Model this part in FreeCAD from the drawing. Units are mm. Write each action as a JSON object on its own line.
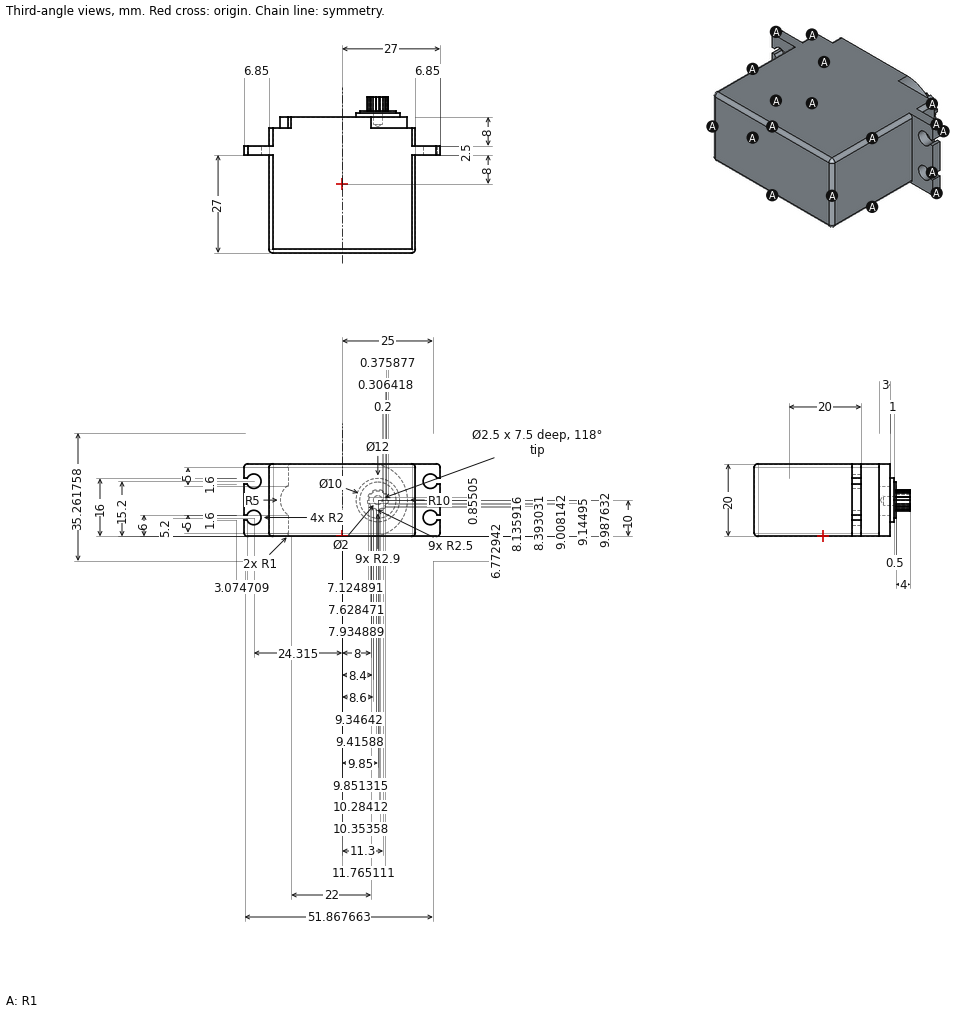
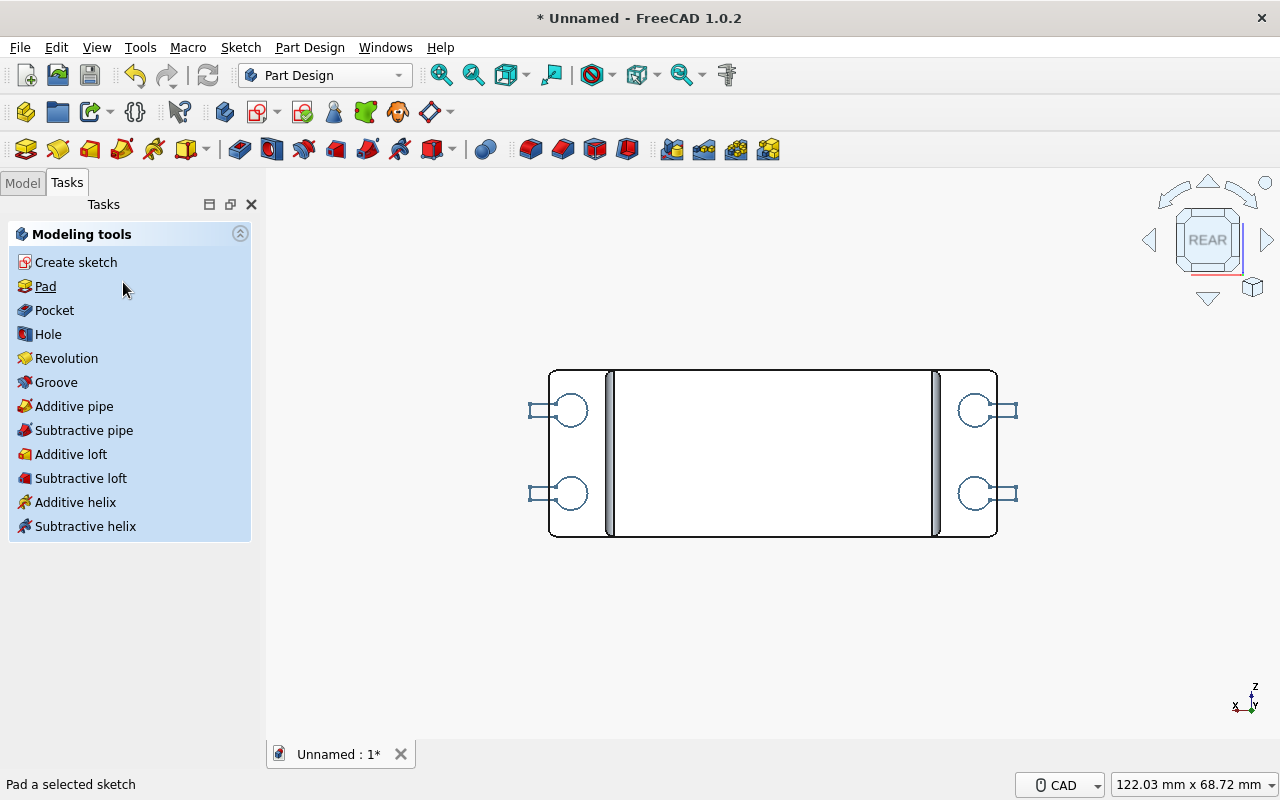
{"action": "left_click", "coordinate": [240, 150]}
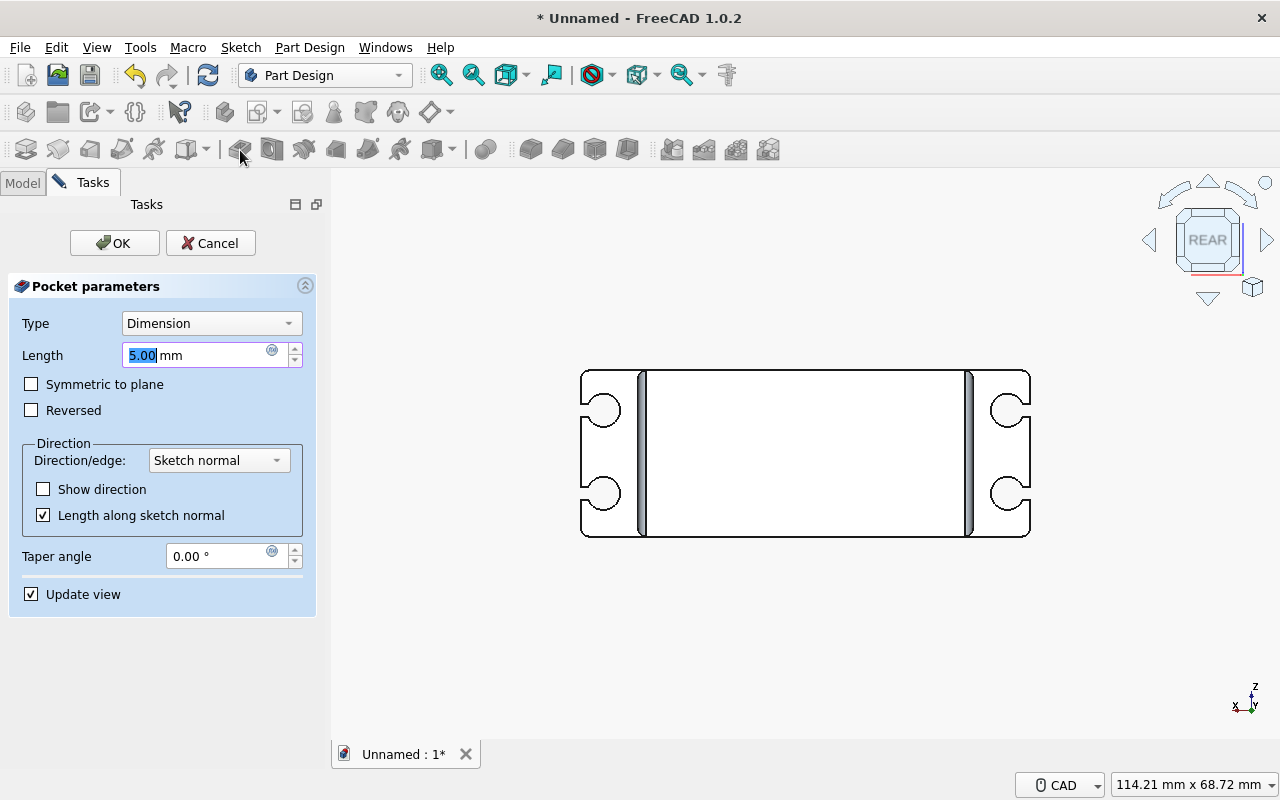
{"action": "type", "text": "20"}
{"action": "key", "text": "Tab"}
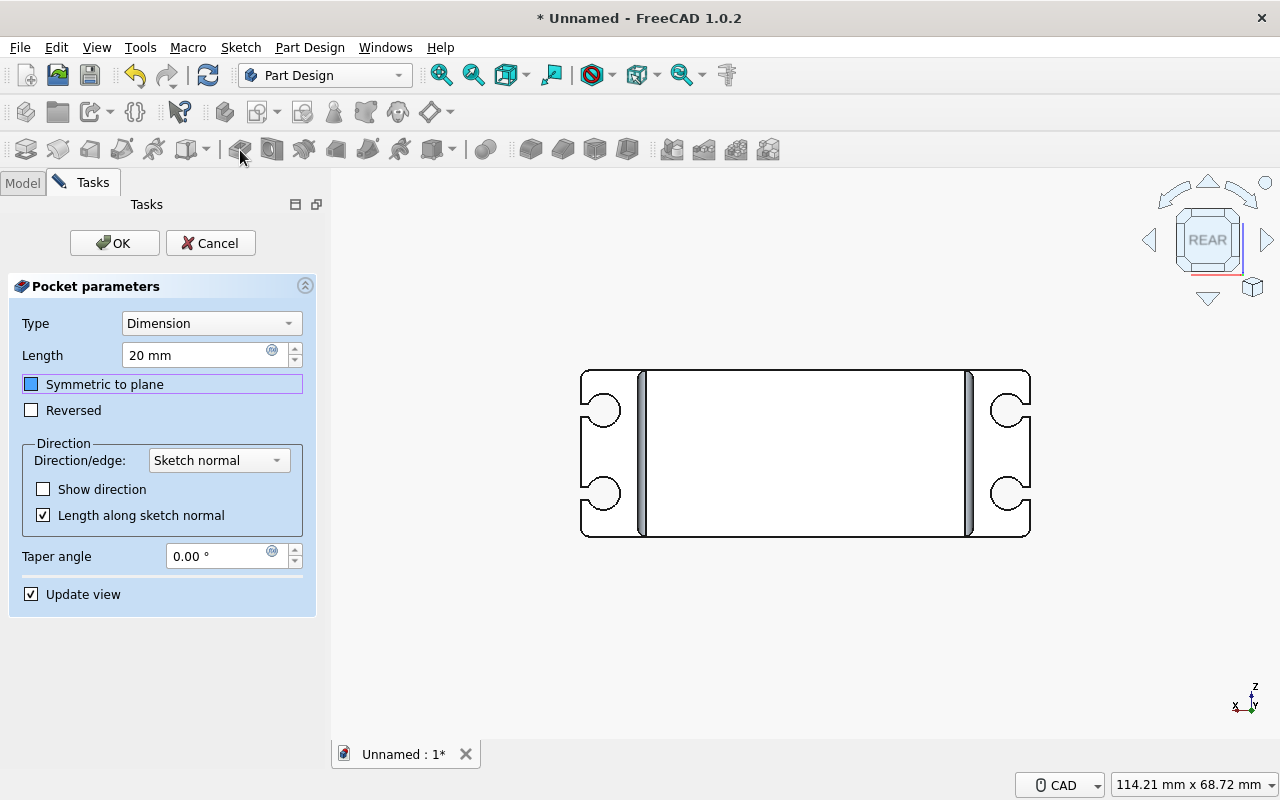
{"action": "left_click", "coordinate": [115, 243]}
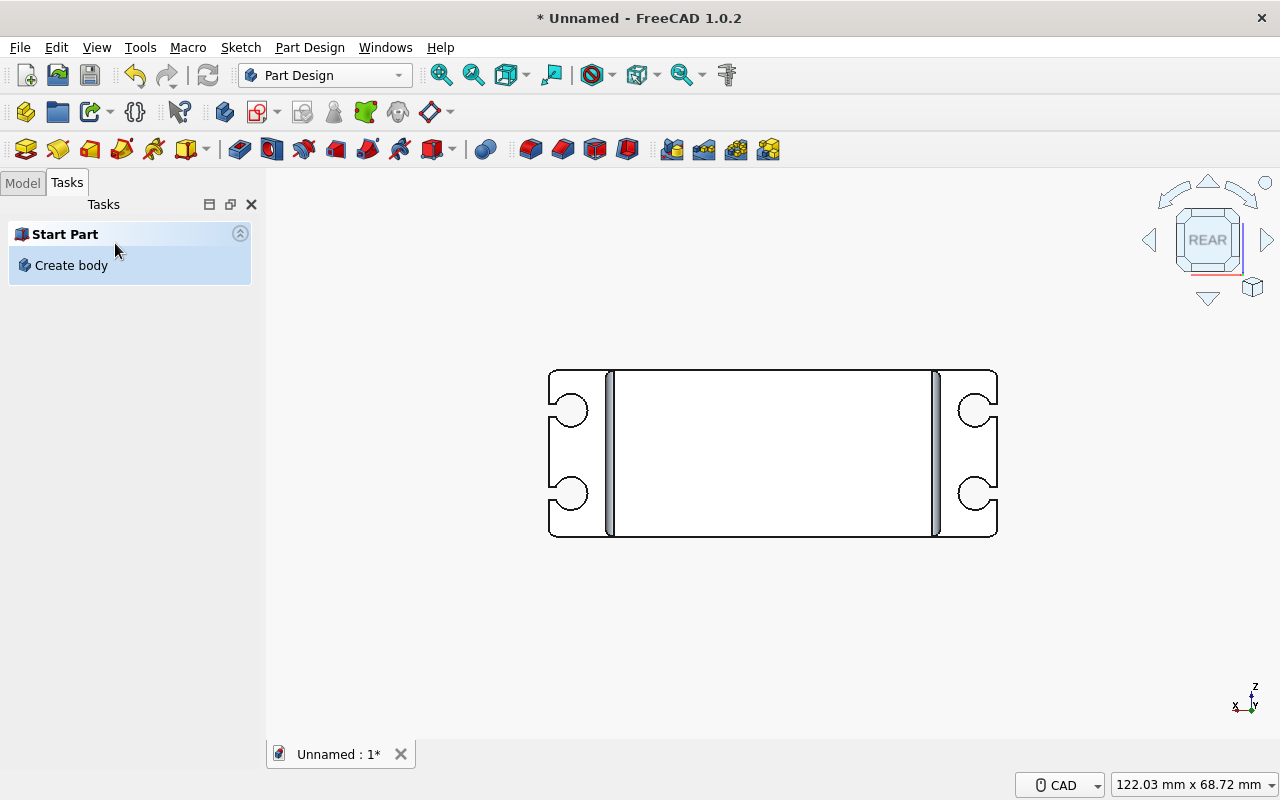
{"action": "left_click", "coordinate": [442, 76]}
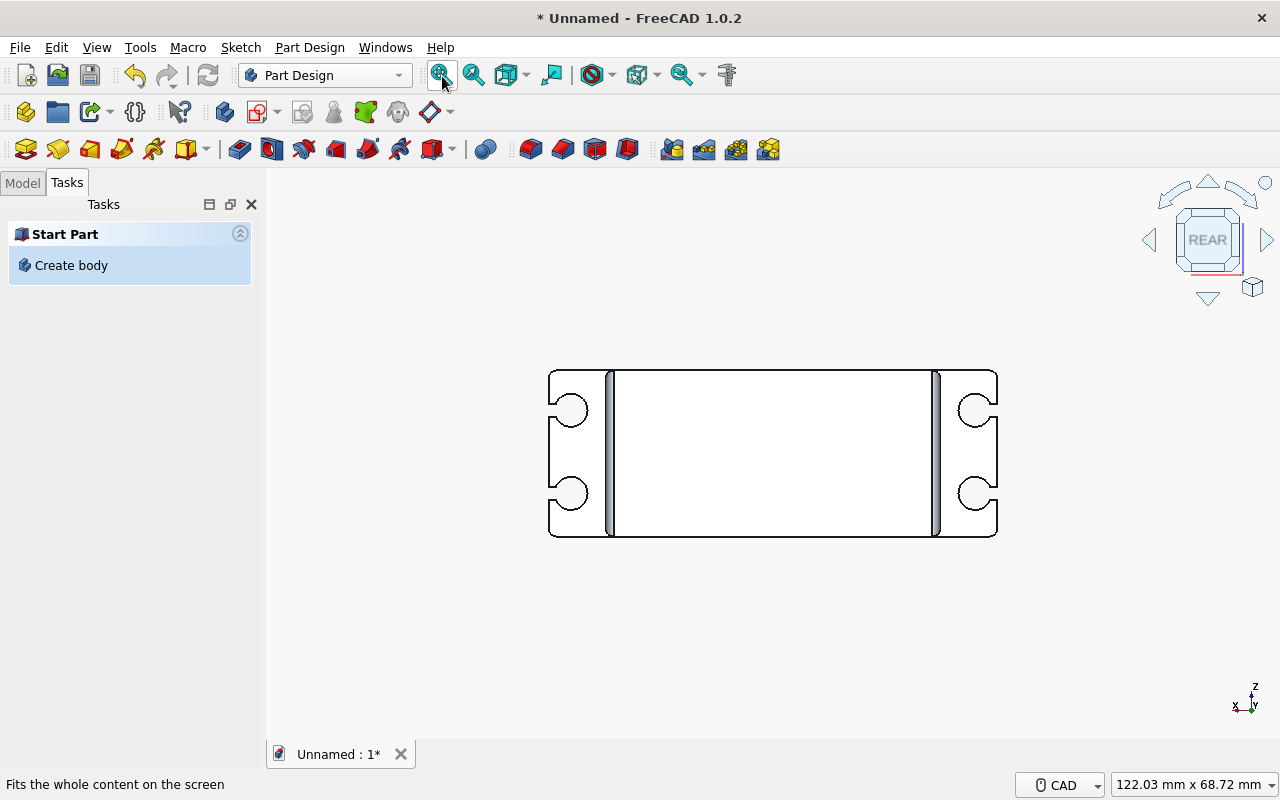
{"action": "left_click", "coordinate": [728, 452]}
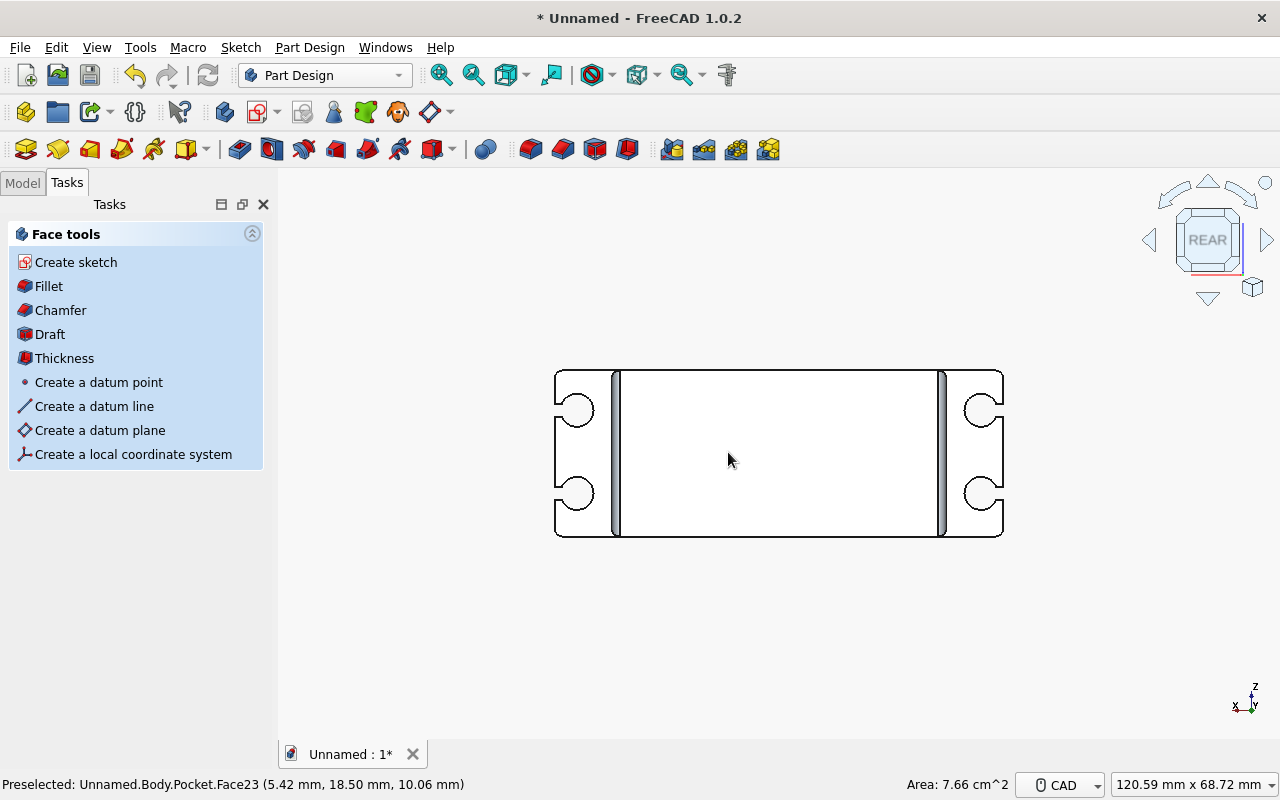
{"action": "left_click", "coordinate": [258, 112]}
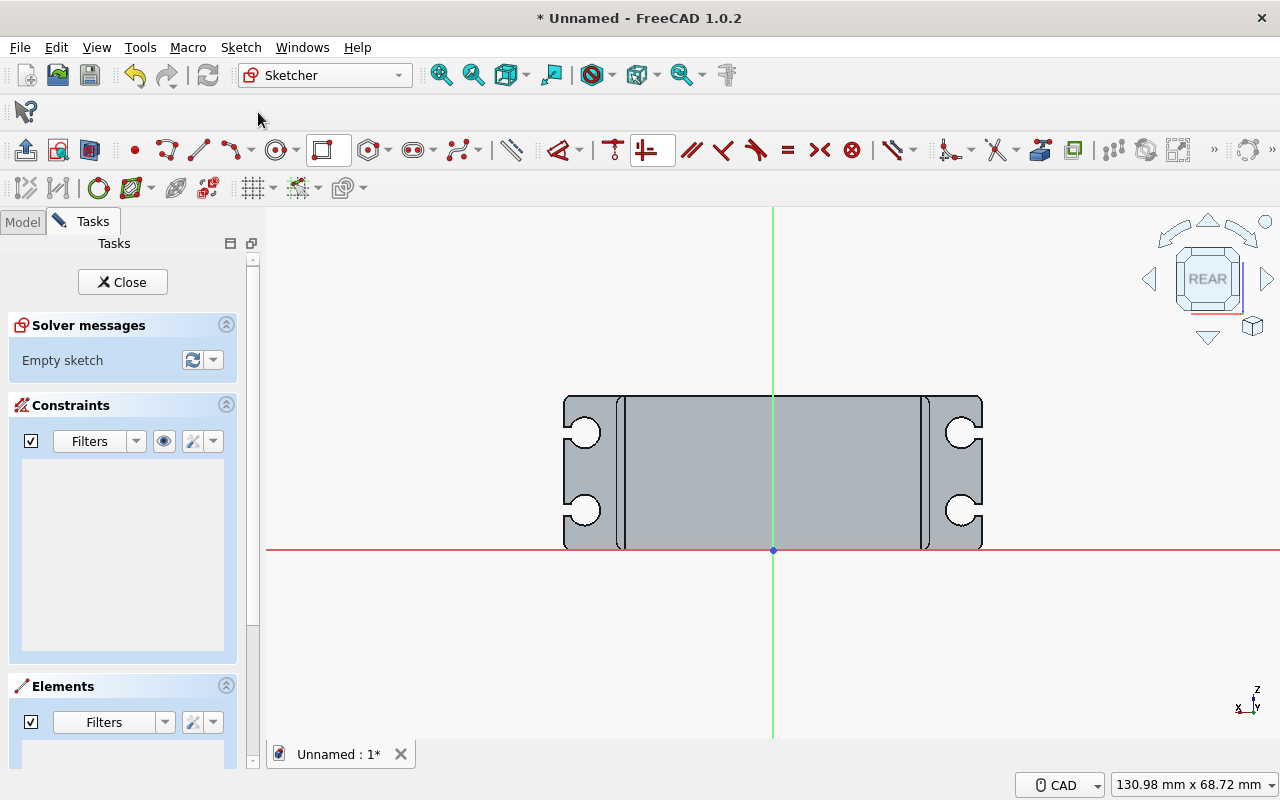
{"action": "left_click", "coordinate": [322, 150]}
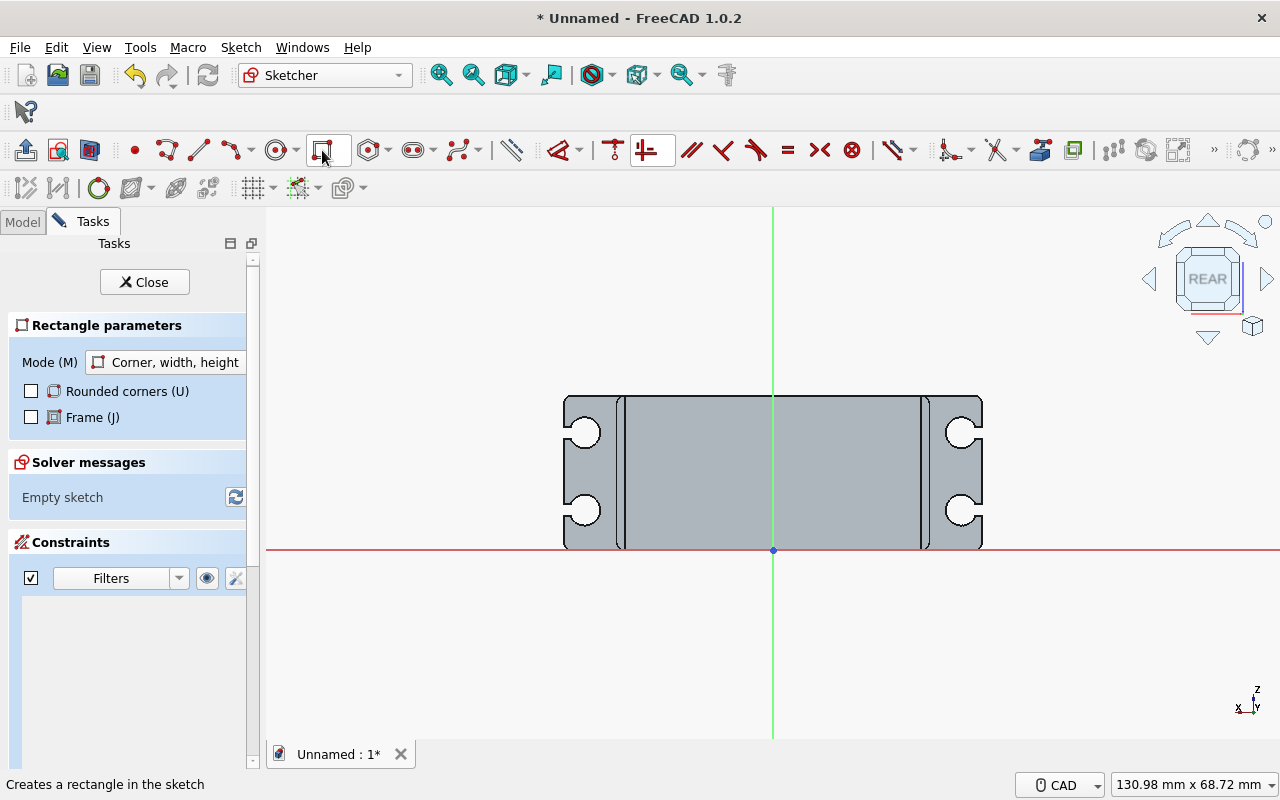
{"action": "left_click", "coordinate": [579, 330]}
{"action": "mouse_move", "coordinate": [981, 603]}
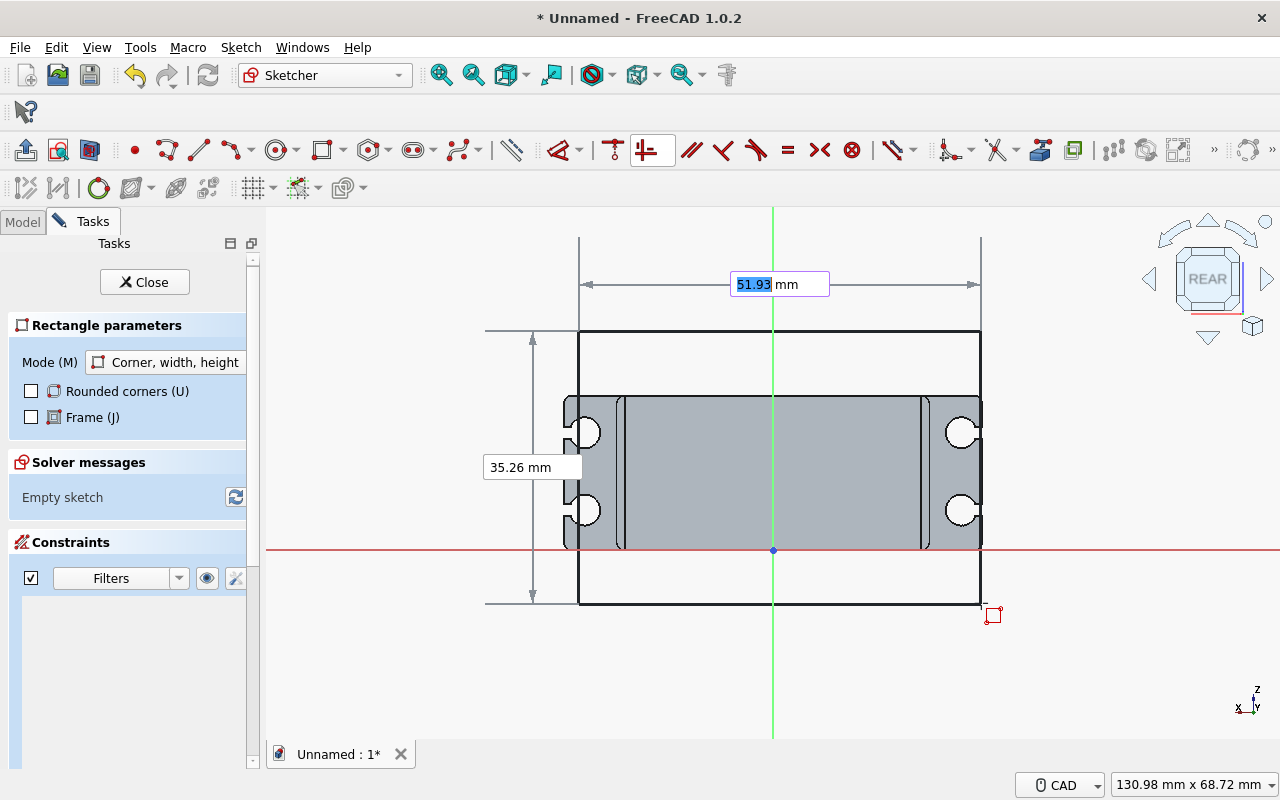
{"action": "type", "text": "51.867663"}
{"action": "key", "text": "Tab"}
{"action": "type", "text": "35.261758"}
{"action": "key", "text": "Return"}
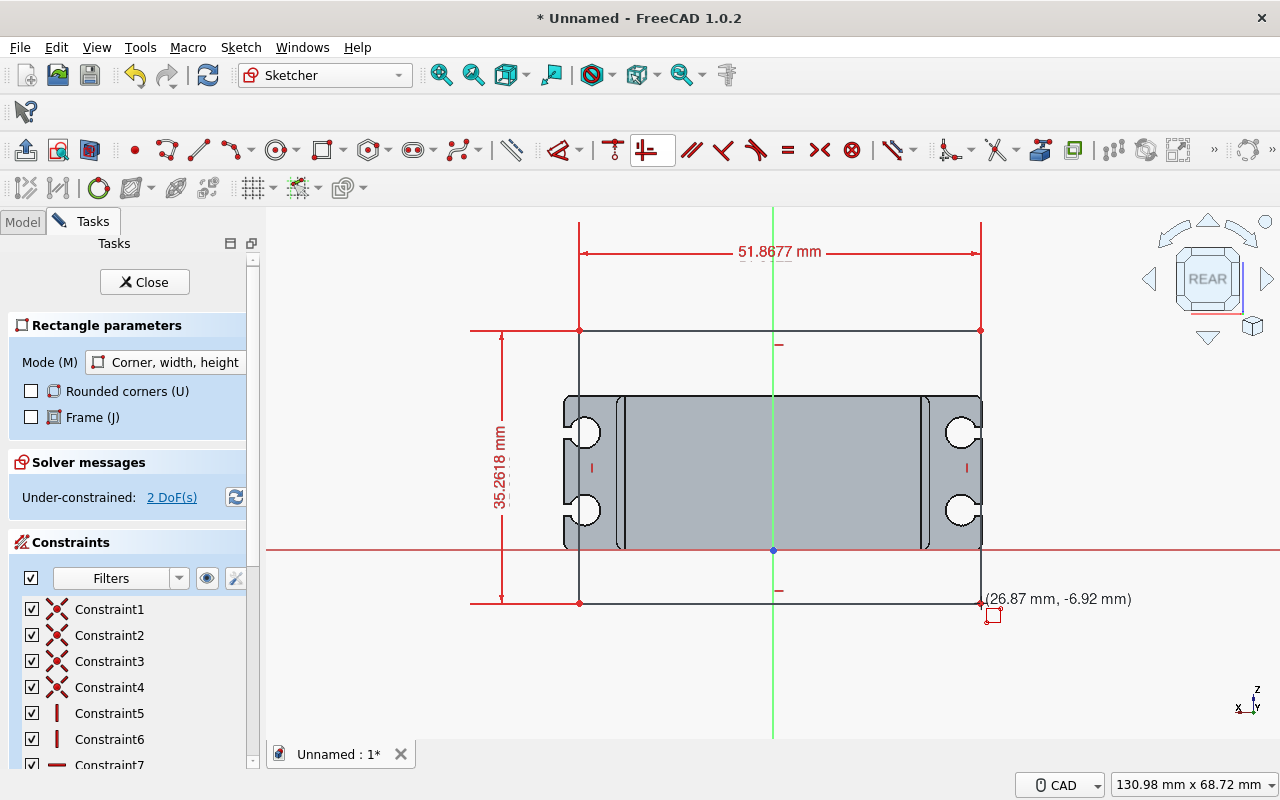
{"action": "left_click", "coordinate": [200, 150]}